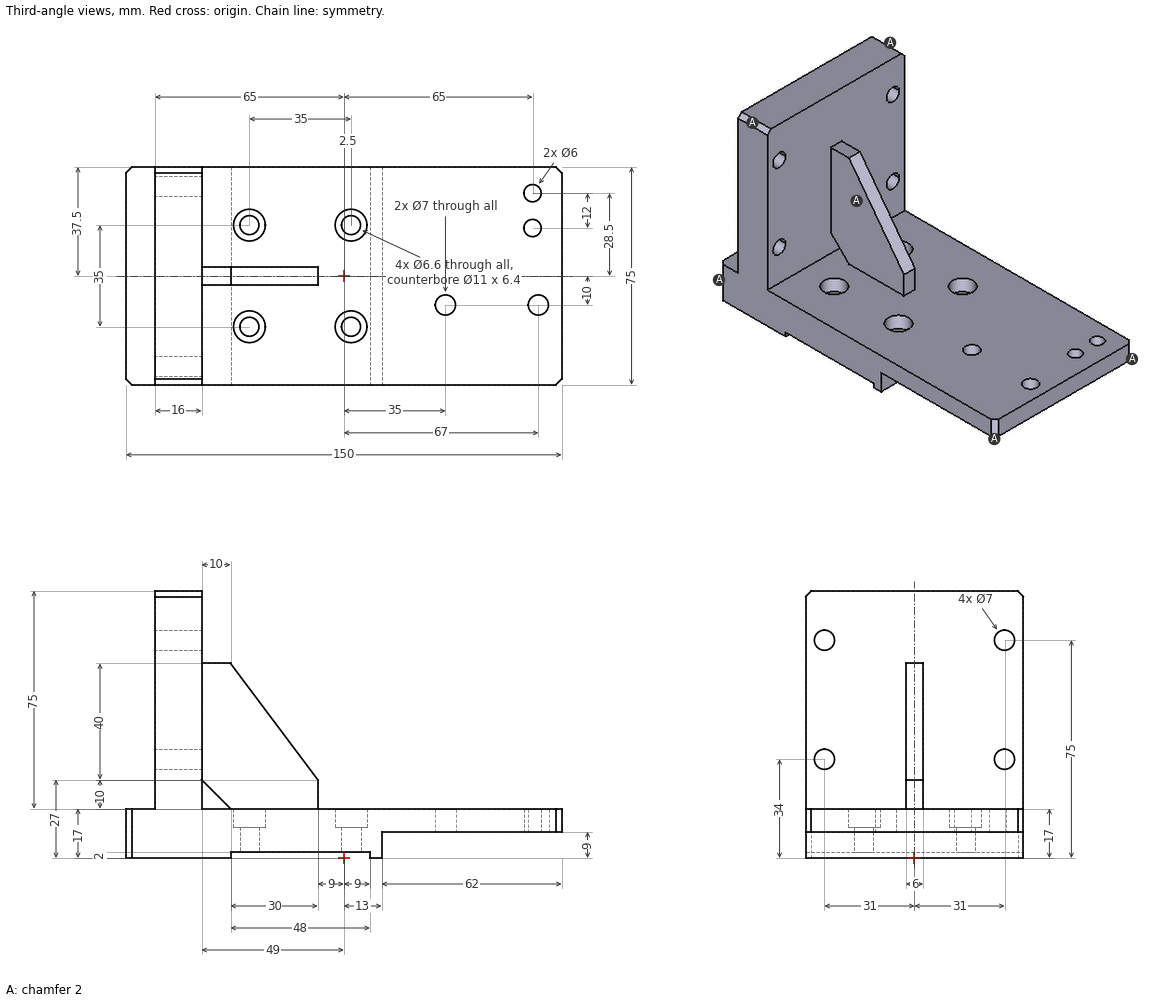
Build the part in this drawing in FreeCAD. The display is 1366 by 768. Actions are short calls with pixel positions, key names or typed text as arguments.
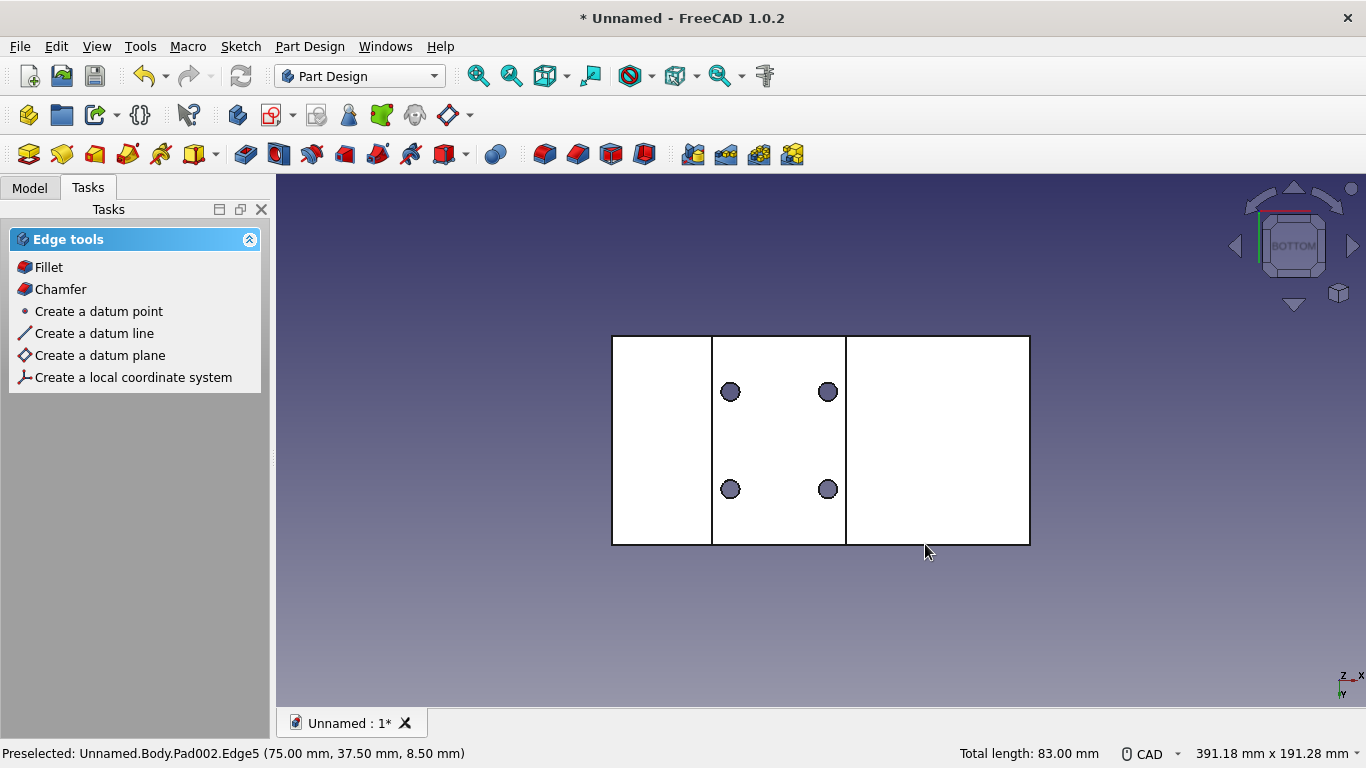
click(479, 76)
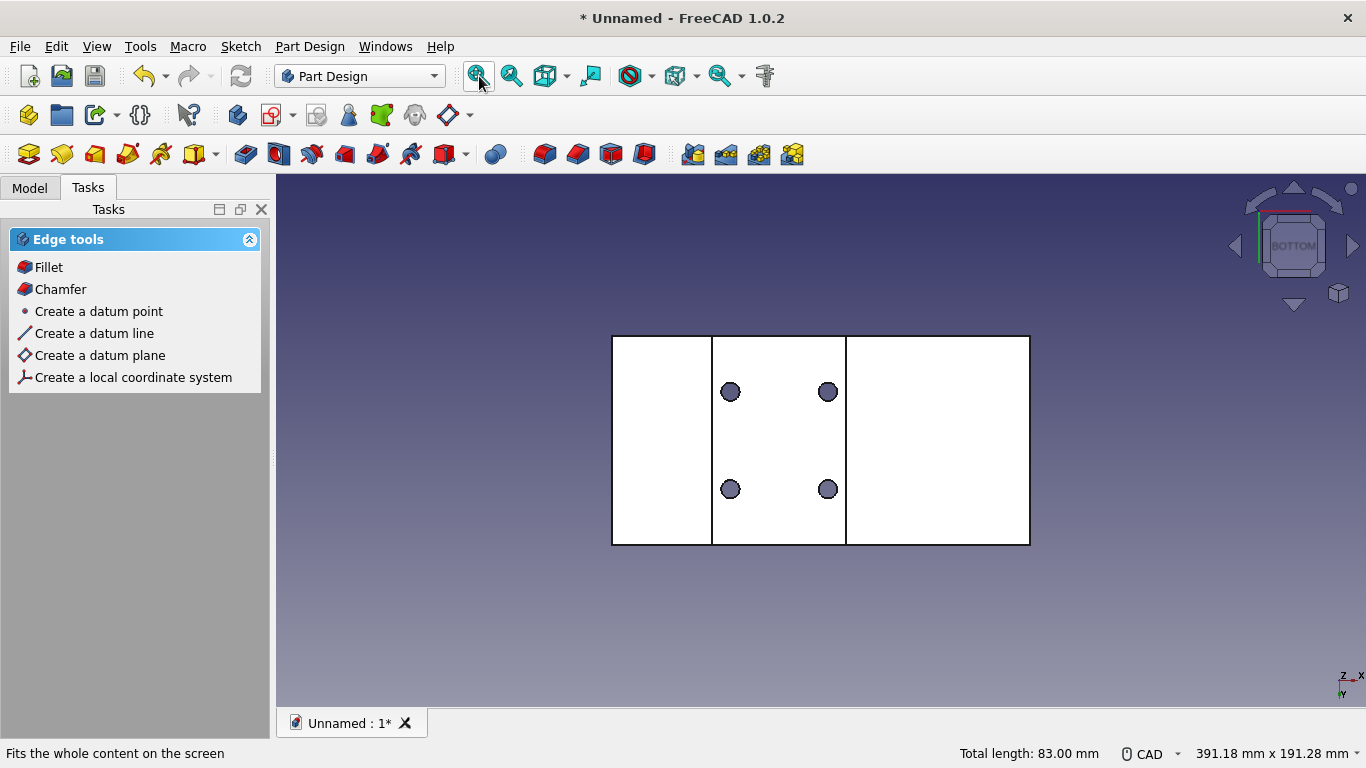
key(4)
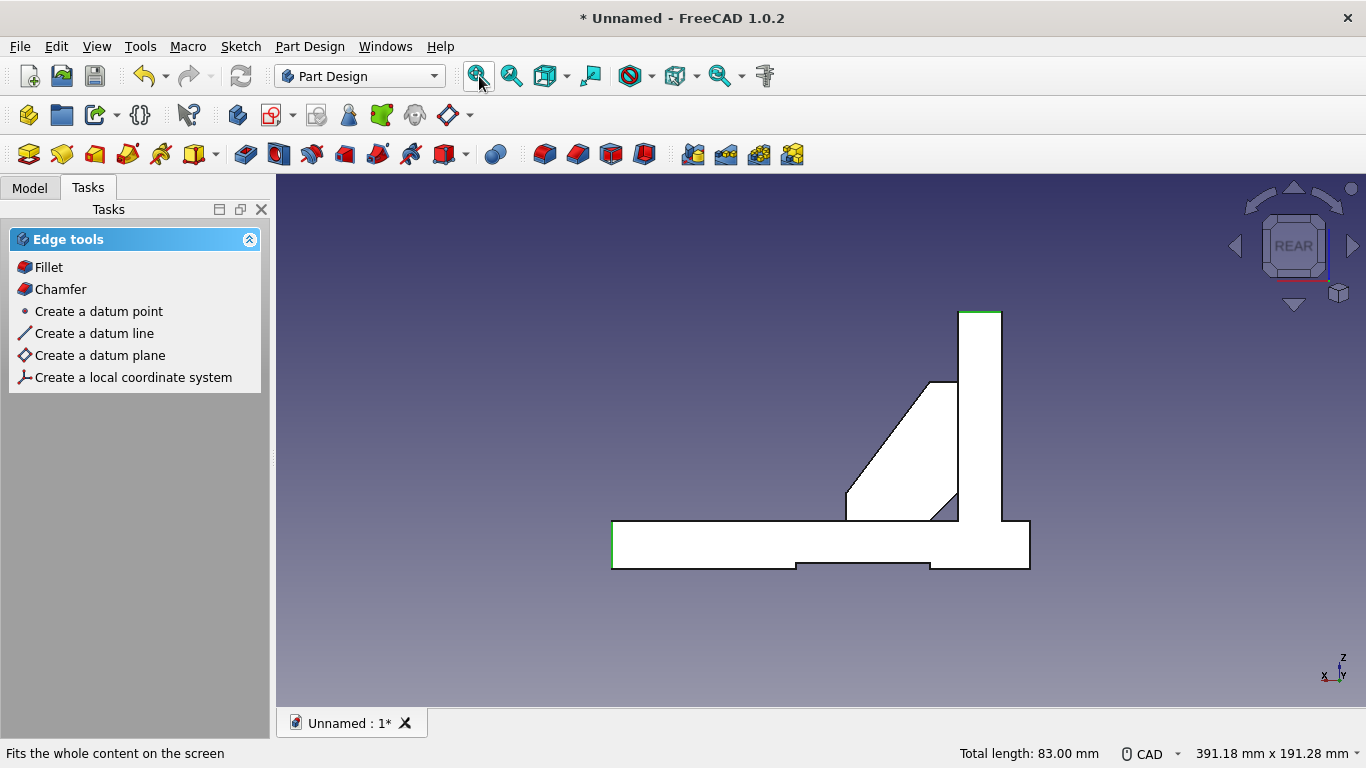
click(1030, 544, ctrl)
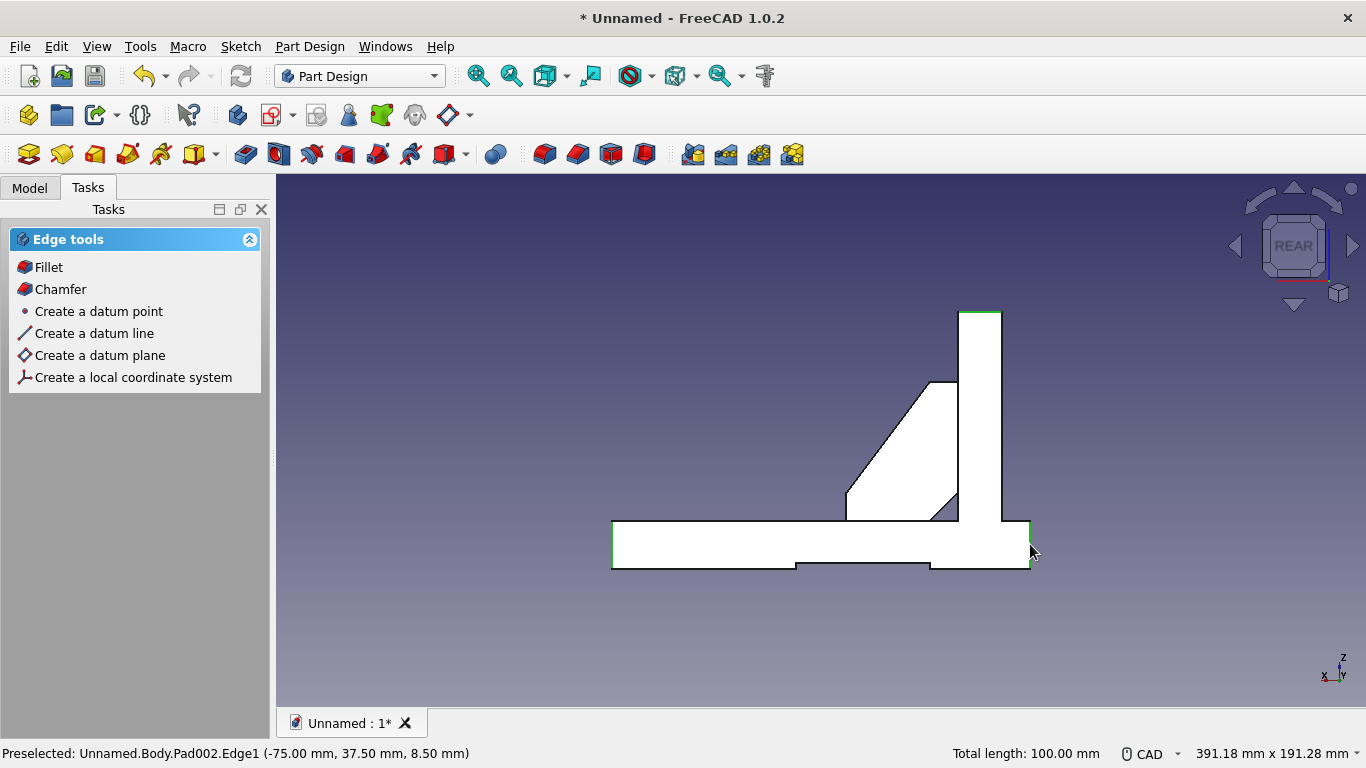
click(578, 154)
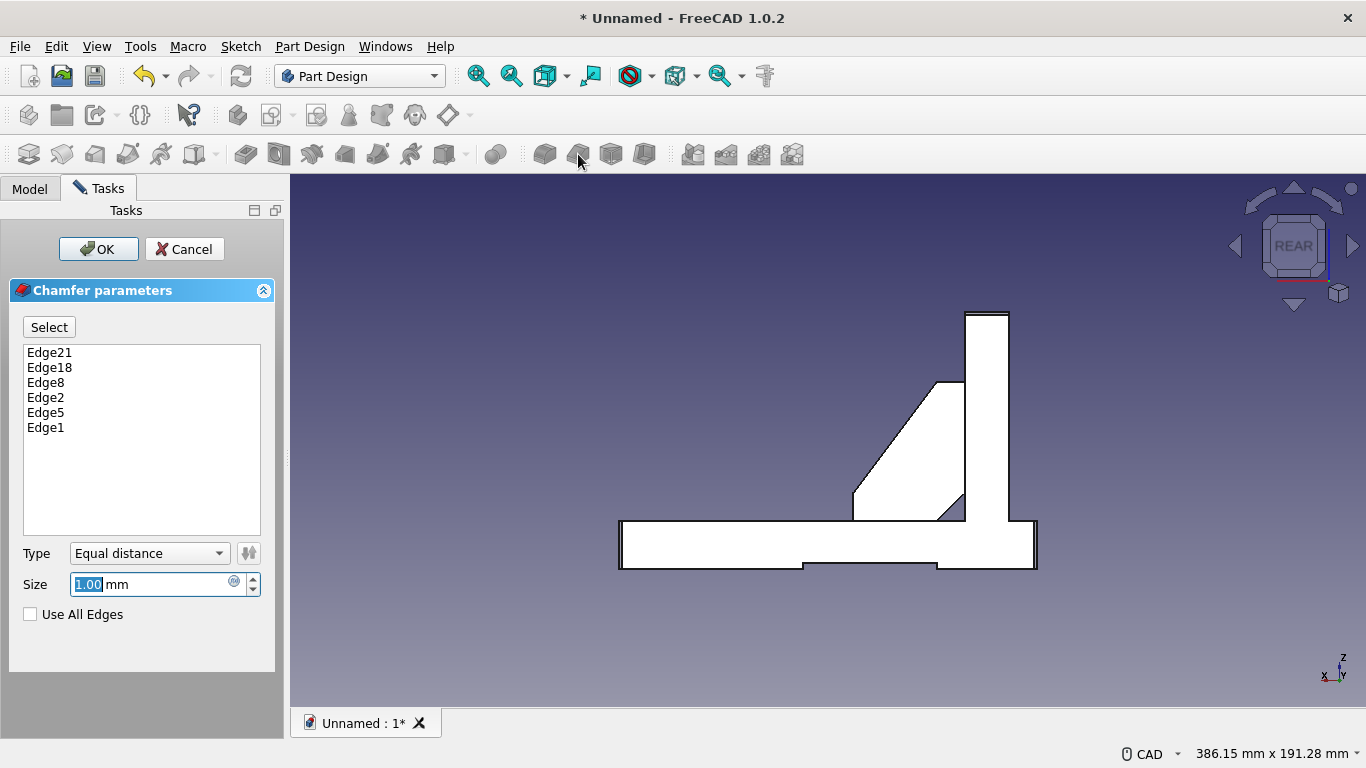
text(2)
key(Tab)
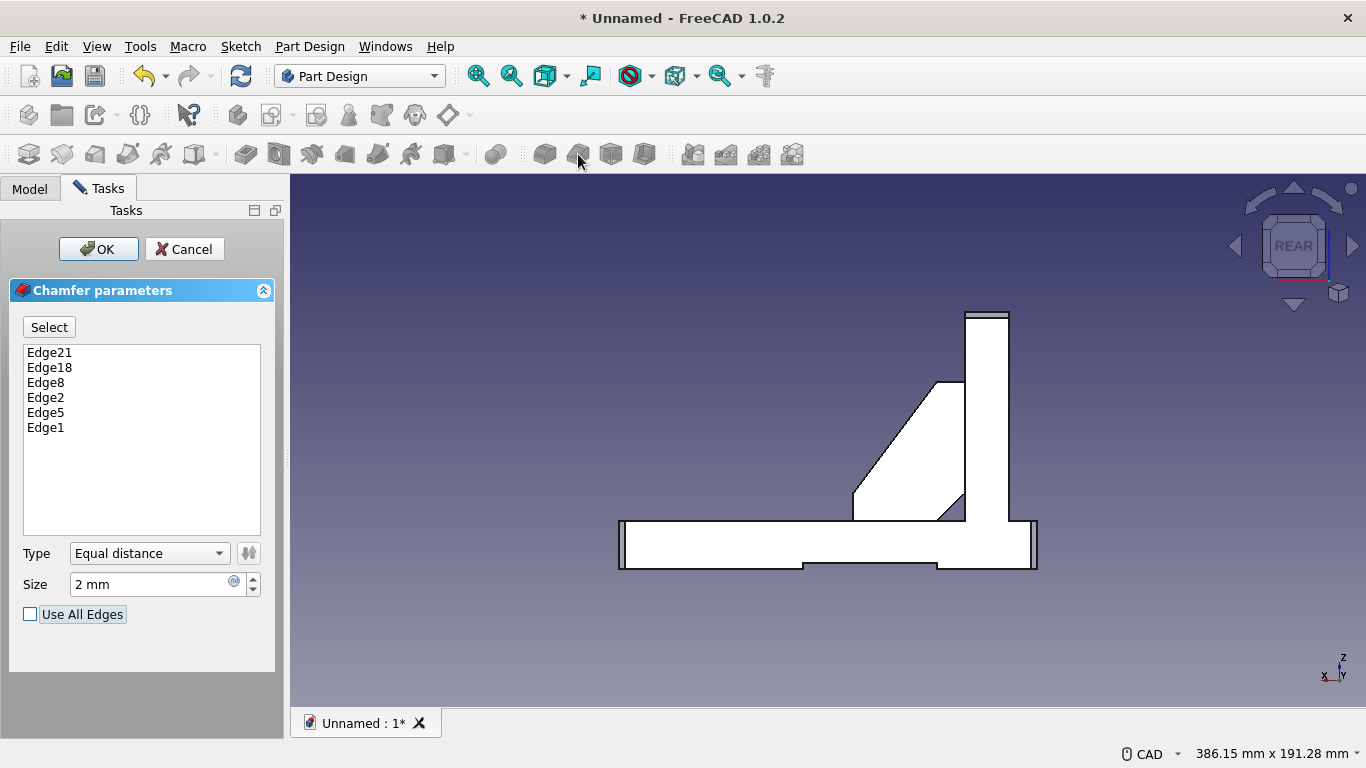
click(99, 249)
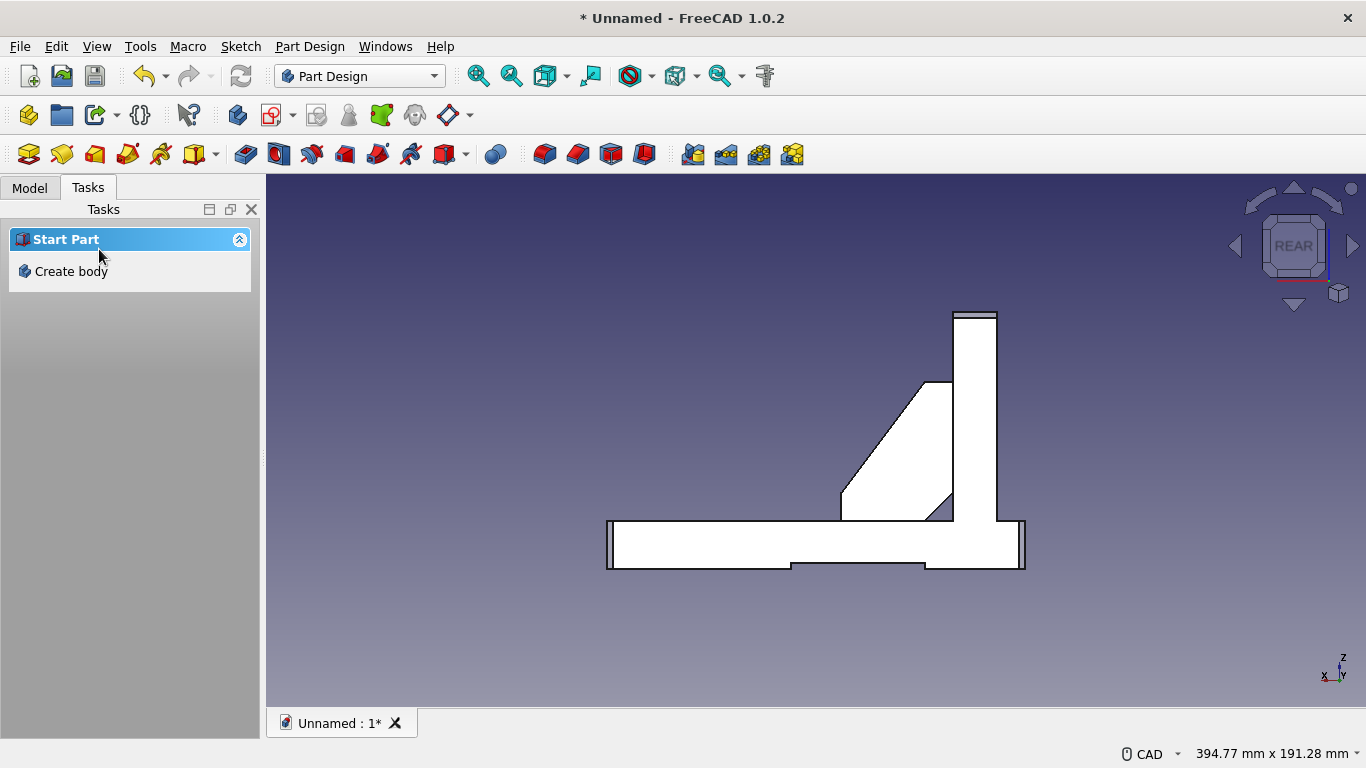
key(0)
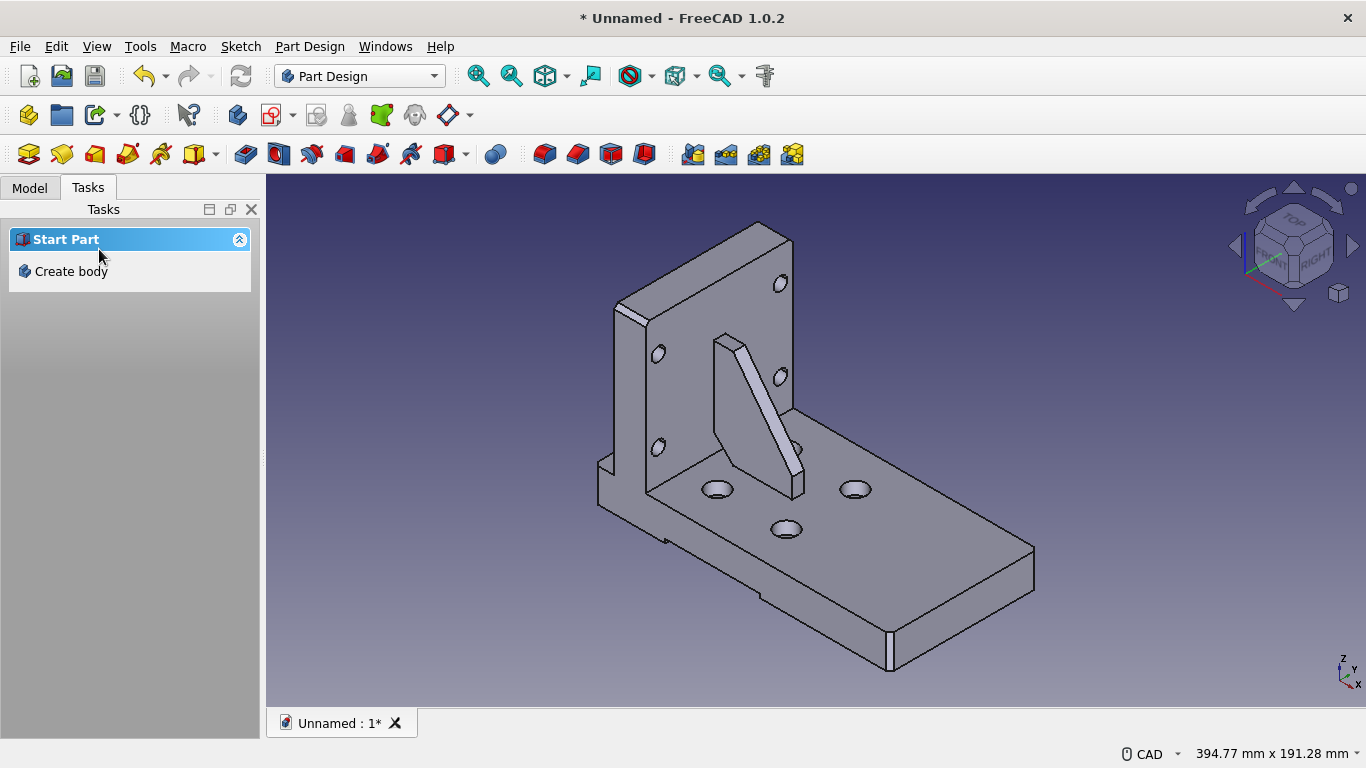
click(865, 643)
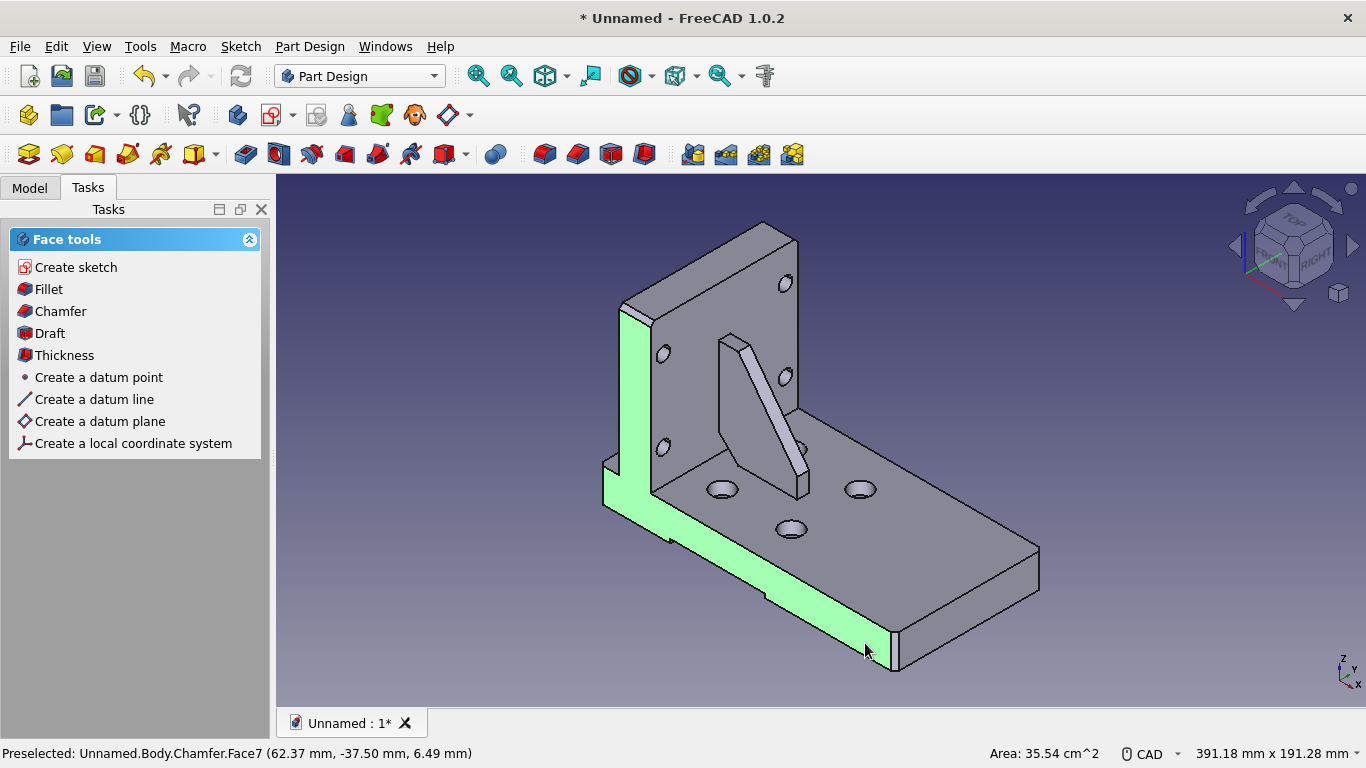
click(270, 116)